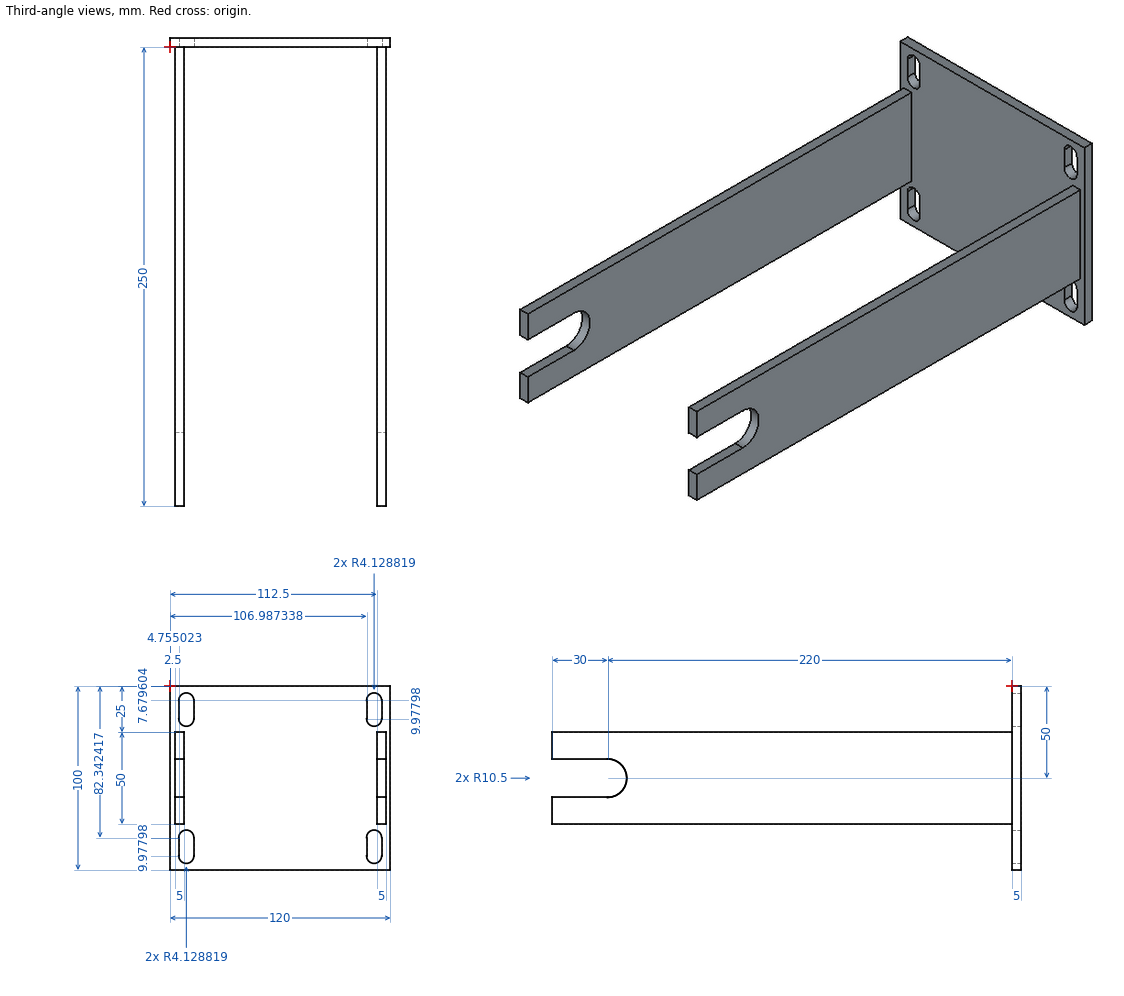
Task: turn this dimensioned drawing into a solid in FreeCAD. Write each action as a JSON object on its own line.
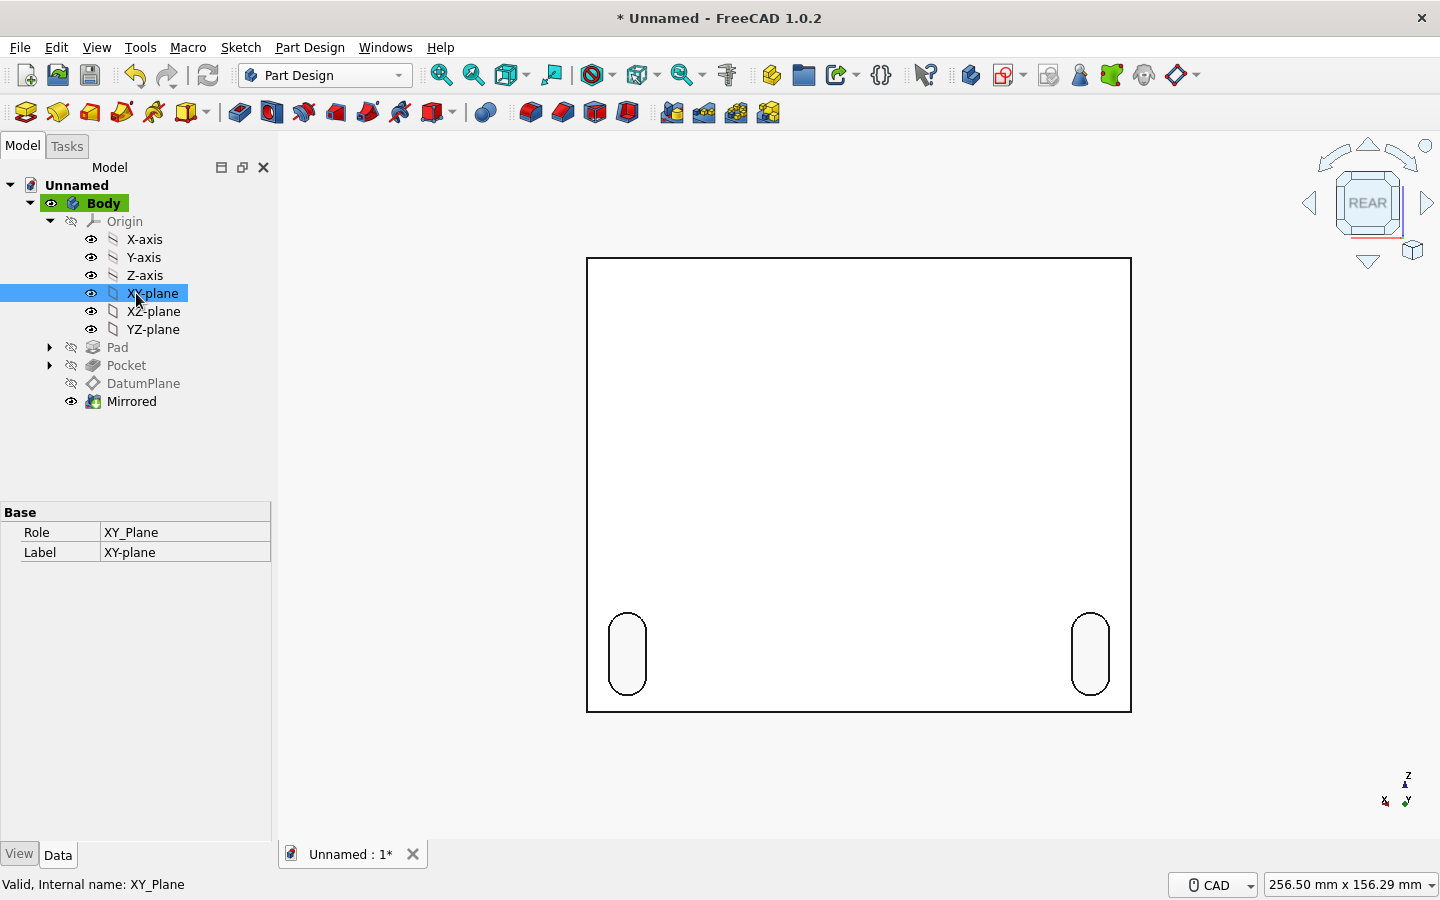
{"action": "left_click", "coordinate": [1176, 76]}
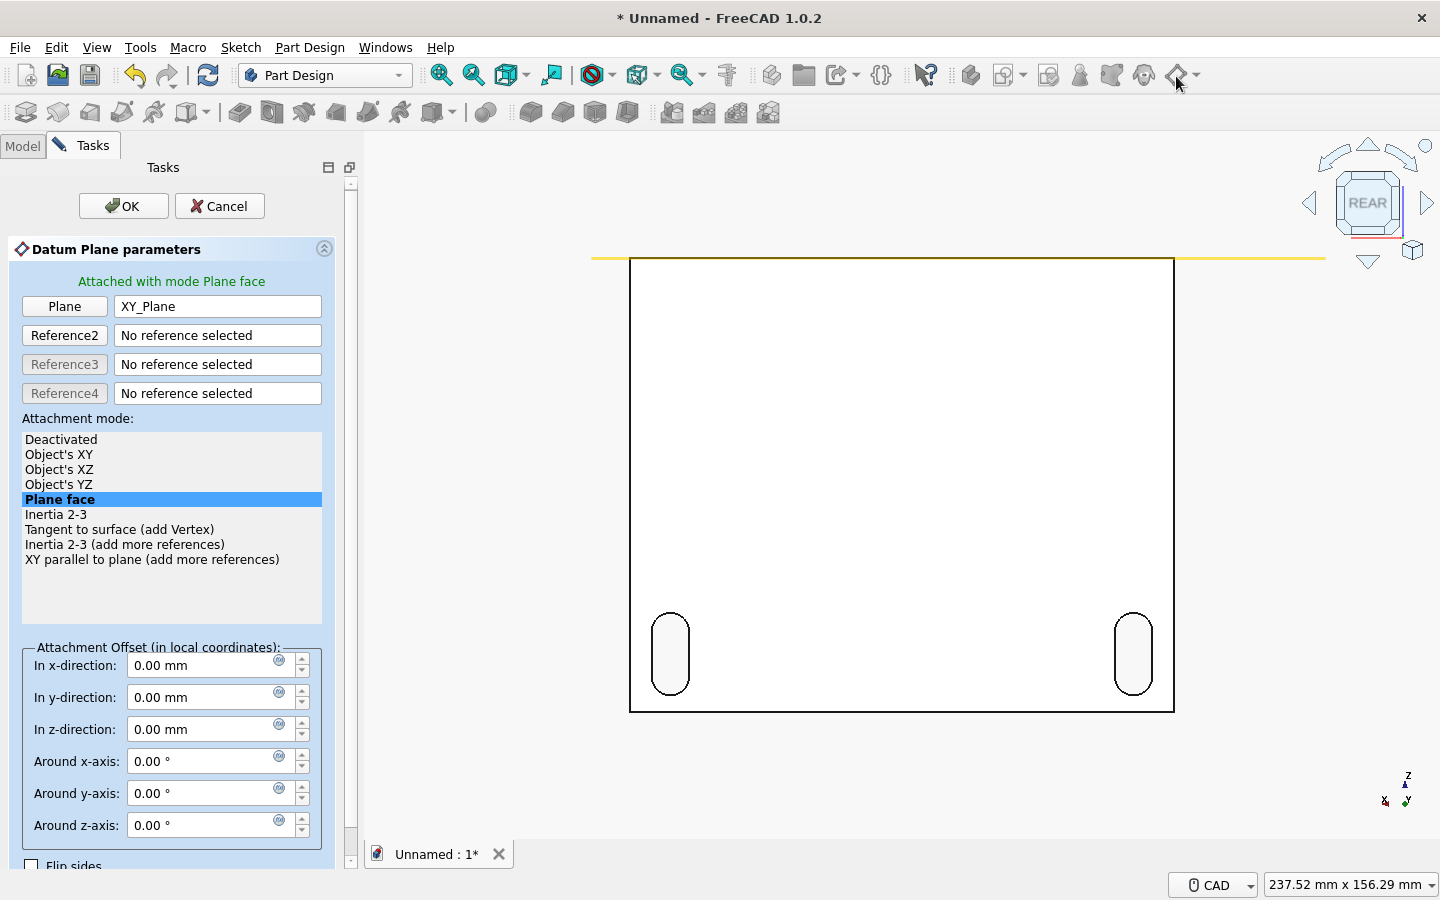
{"action": "triple_click", "coordinate": [210, 729]}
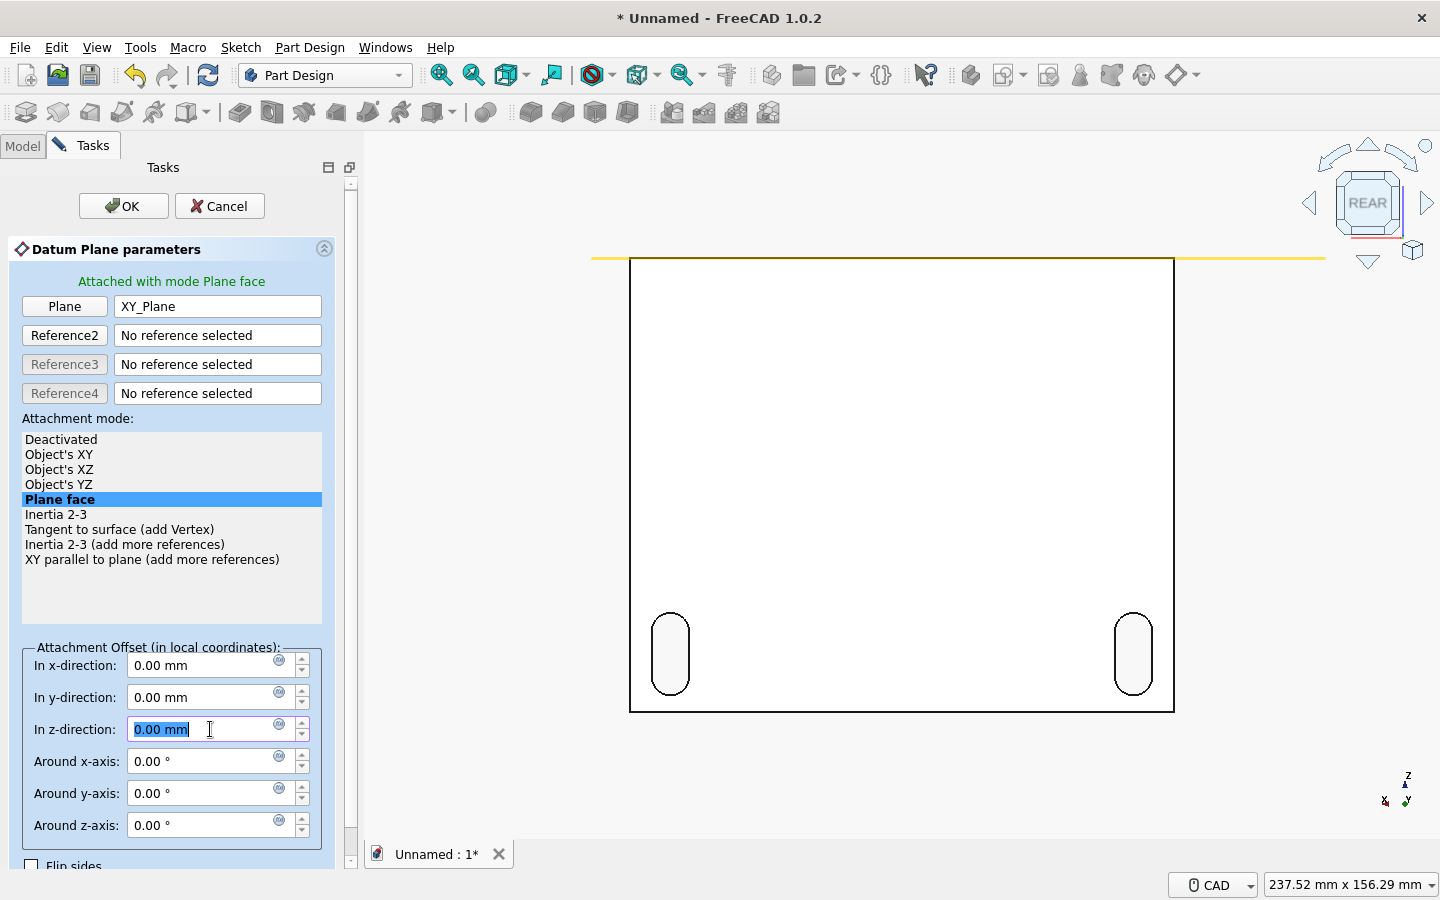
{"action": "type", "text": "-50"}
{"action": "key", "text": "Tab"}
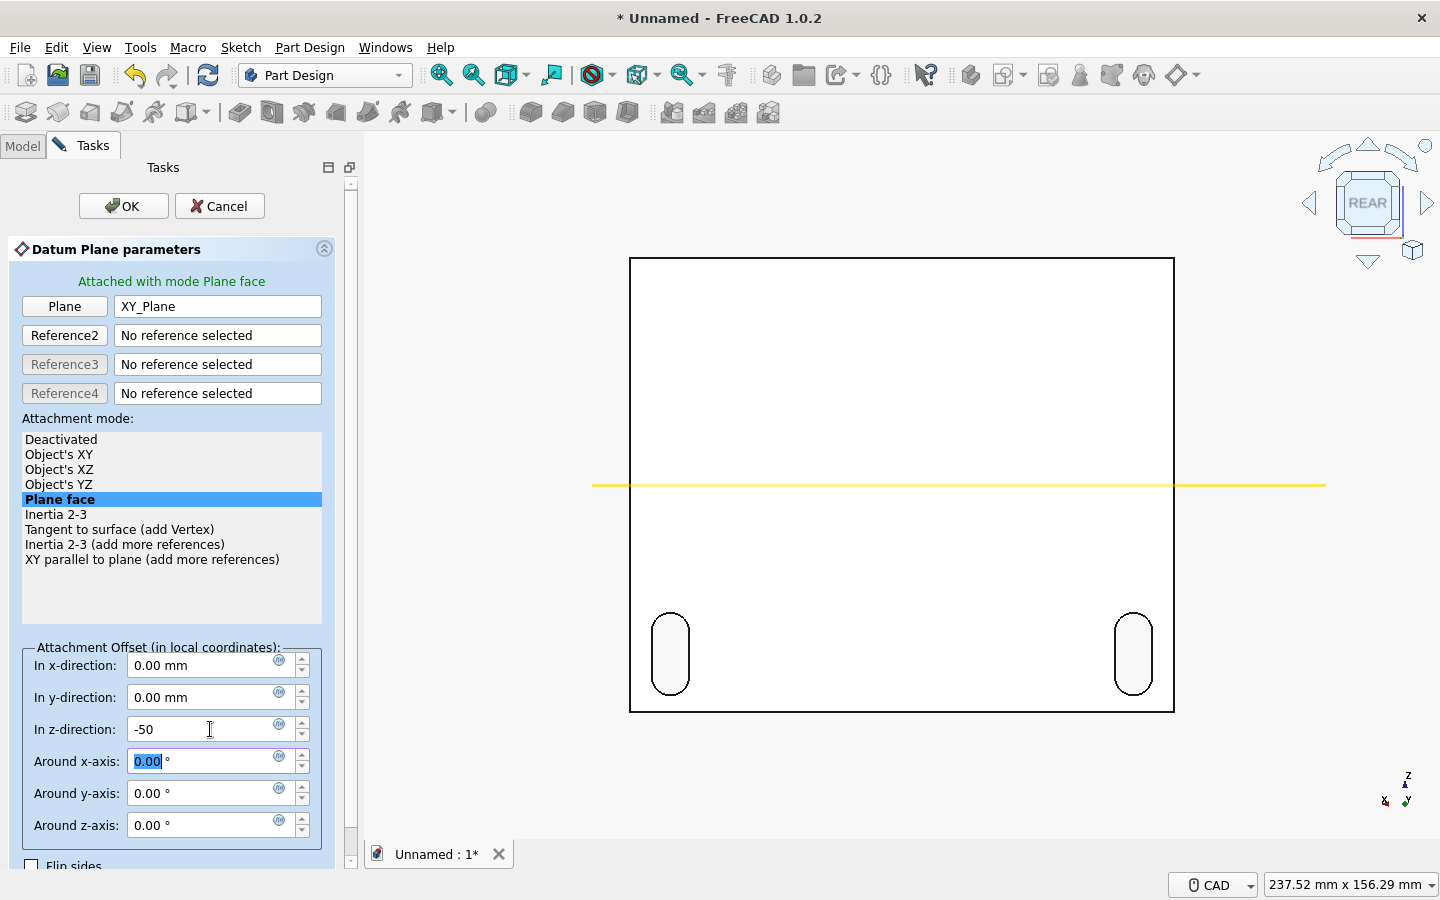
{"action": "left_click", "coordinate": [124, 206]}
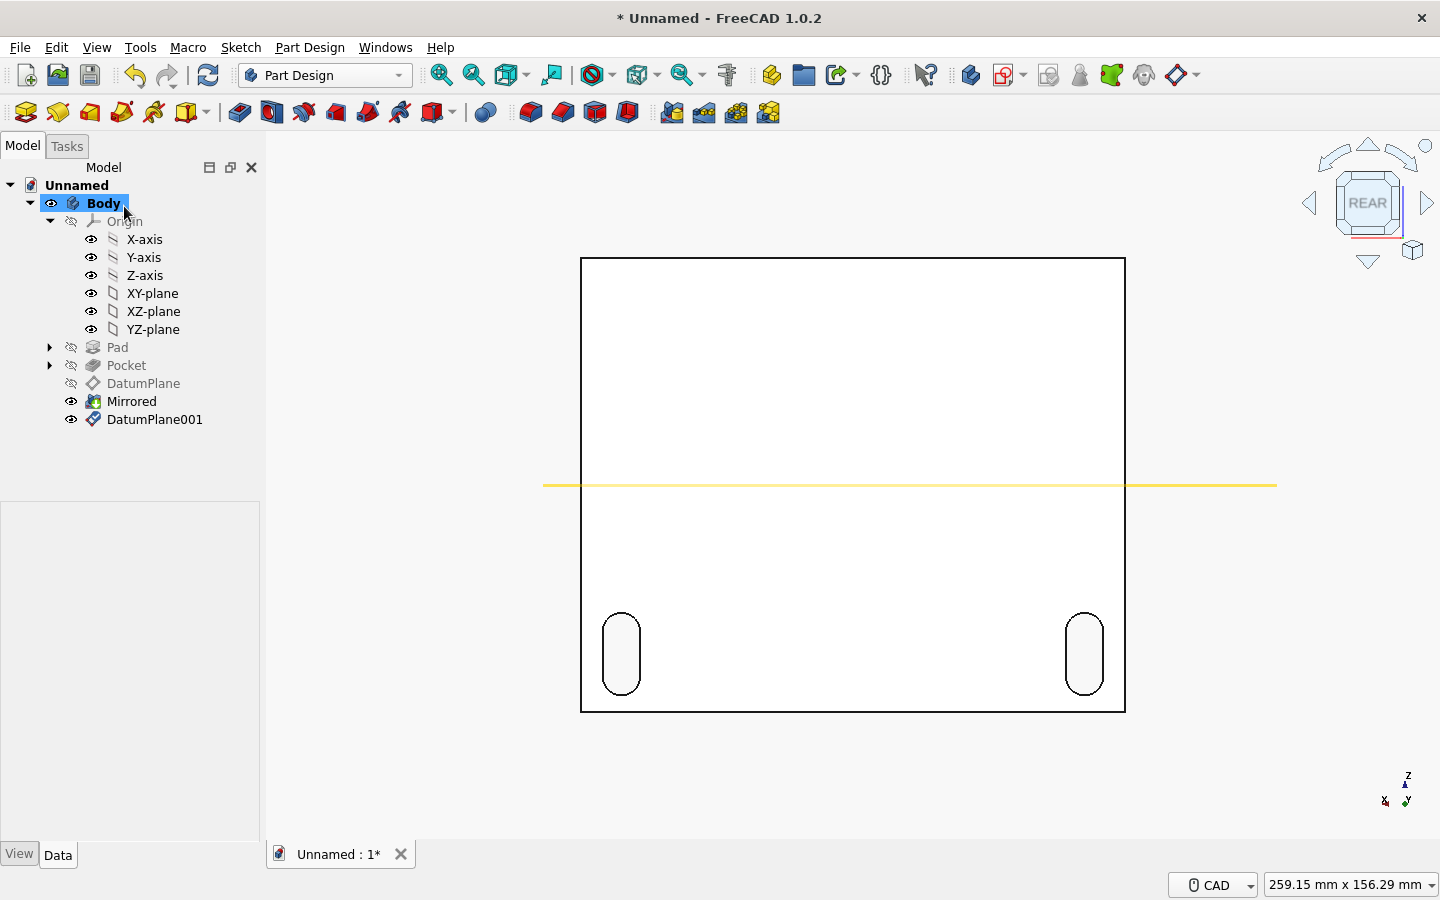
{"action": "left_click", "coordinate": [116, 365]}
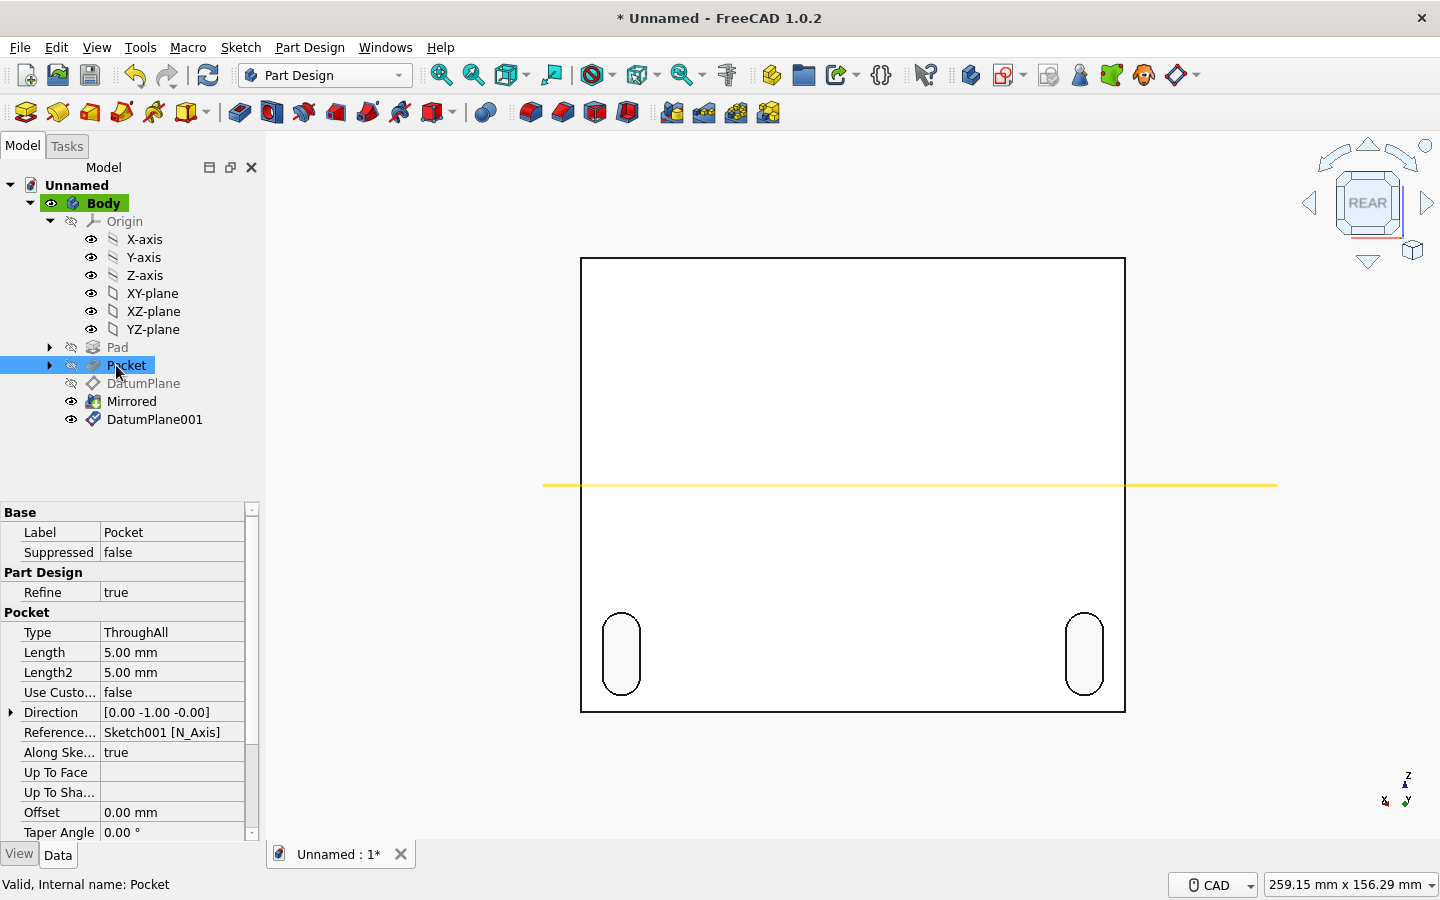
{"action": "left_click", "coordinate": [672, 112]}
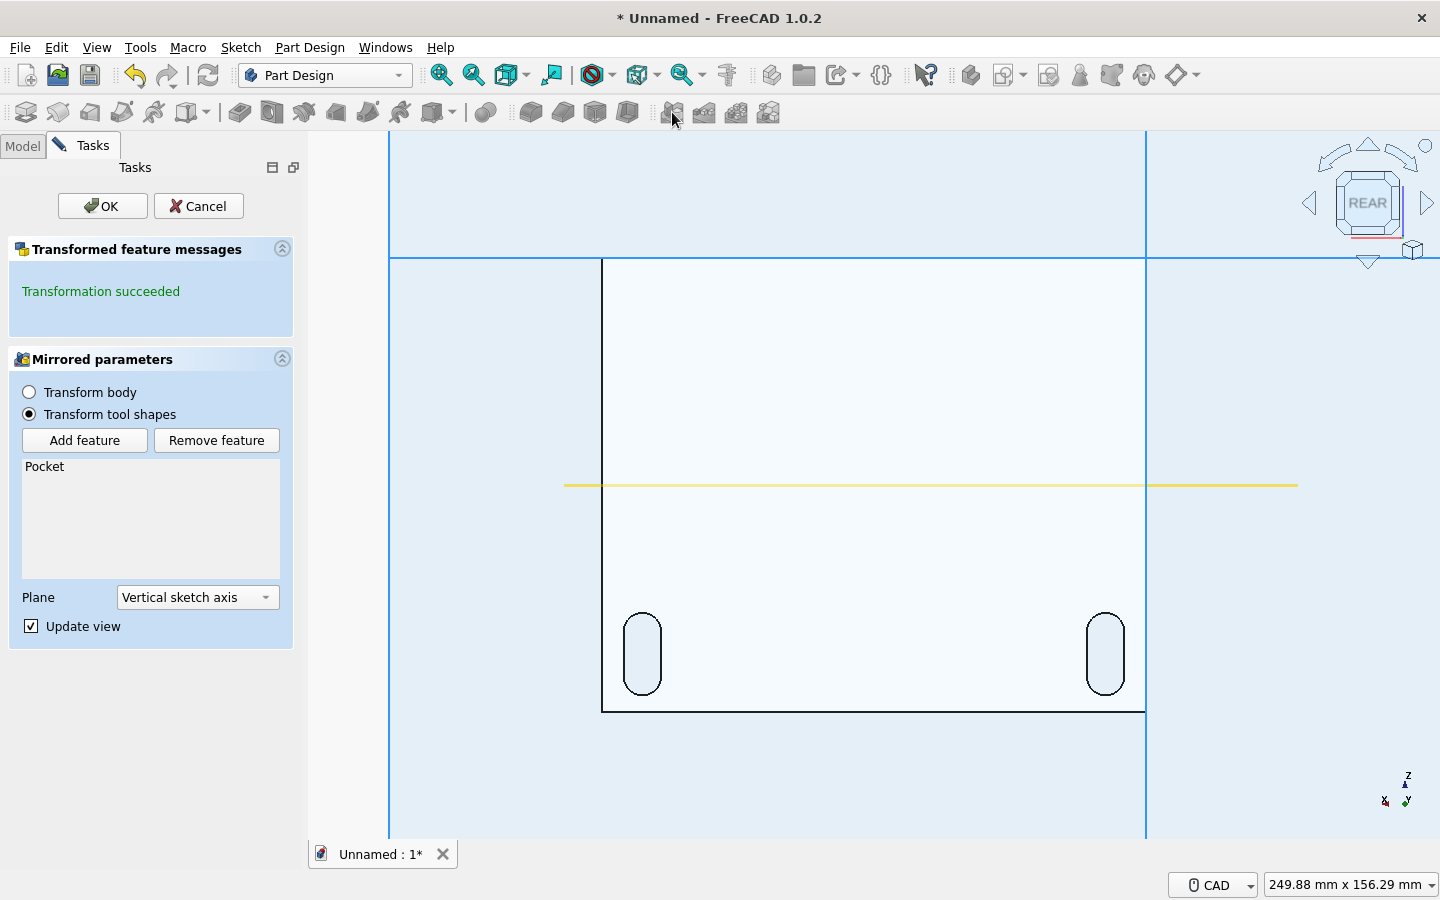
{"action": "left_click", "coordinate": [198, 598]}